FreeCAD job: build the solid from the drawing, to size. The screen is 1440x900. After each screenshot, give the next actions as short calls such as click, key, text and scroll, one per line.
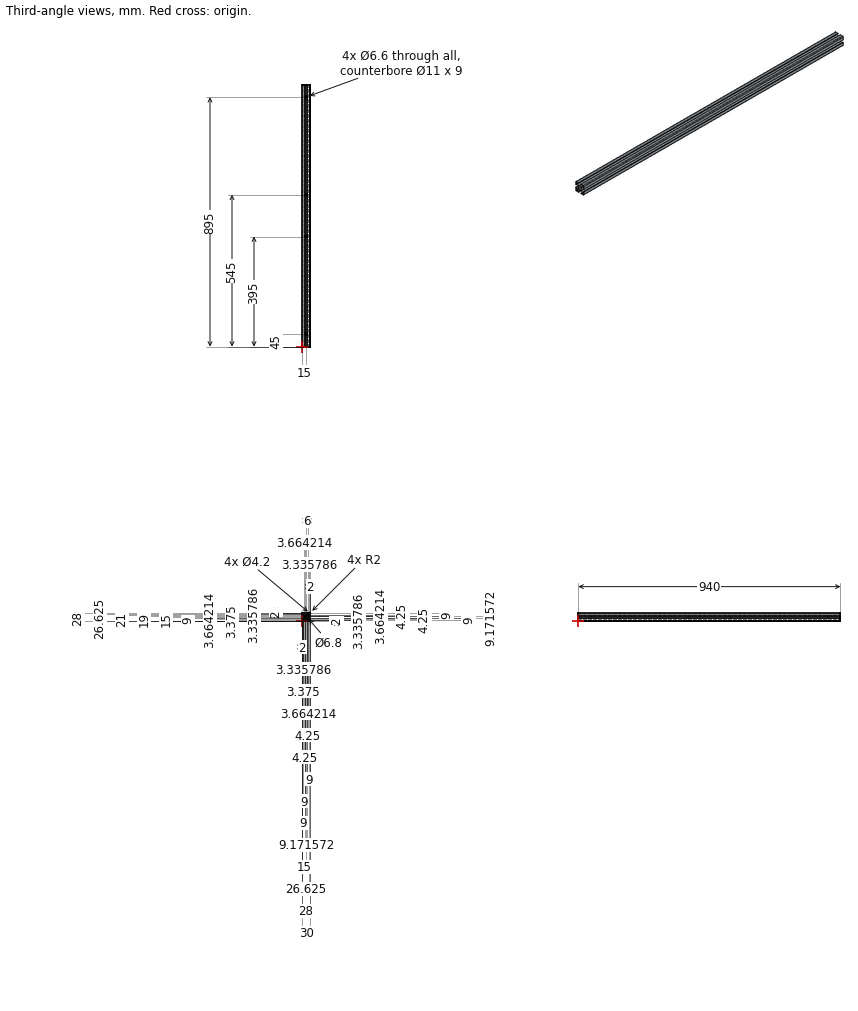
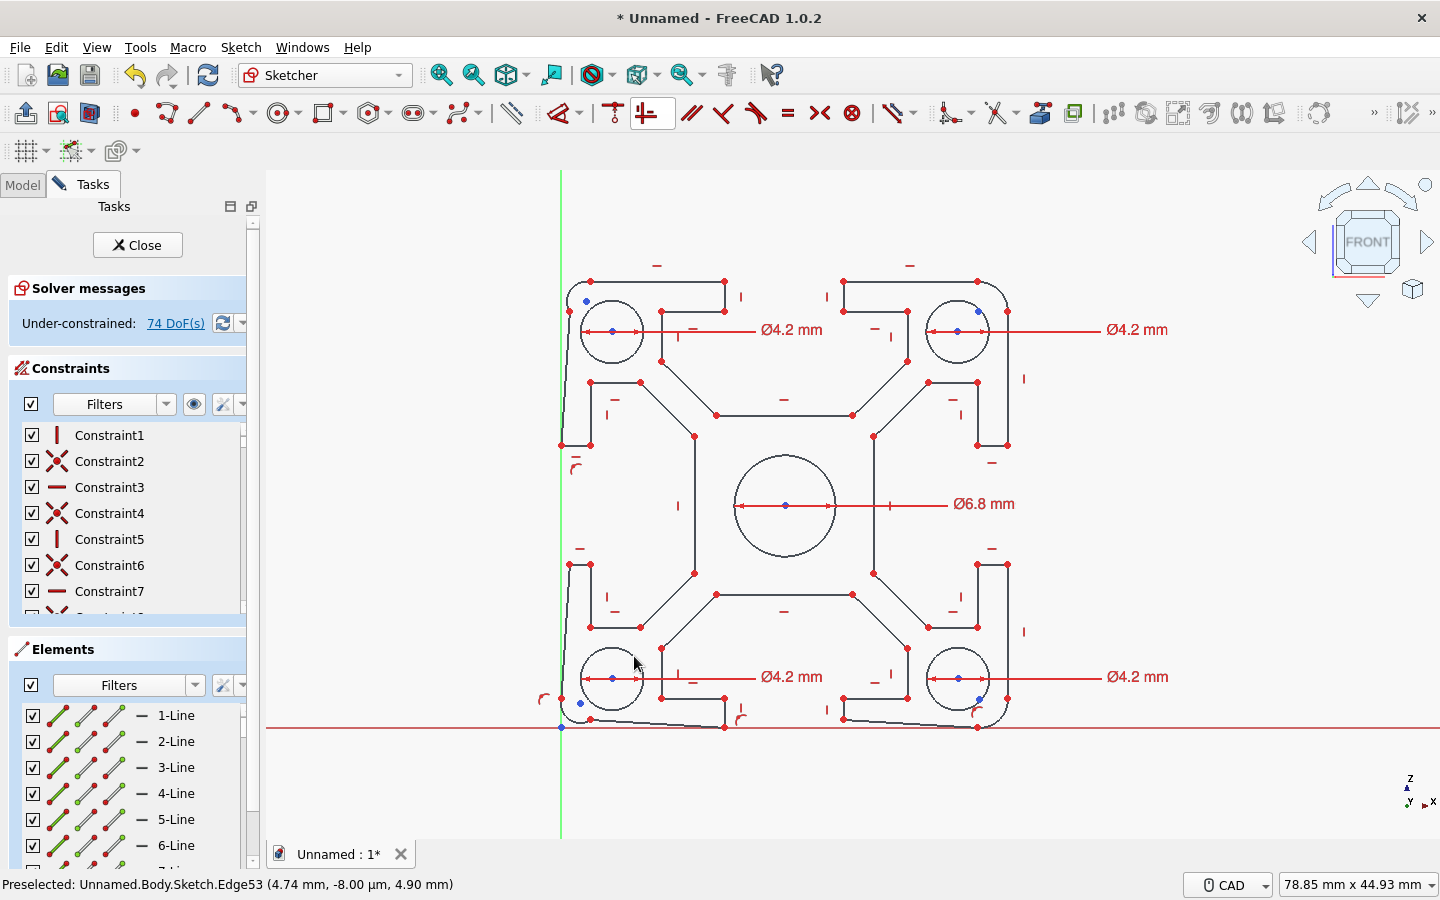
click(1008, 352)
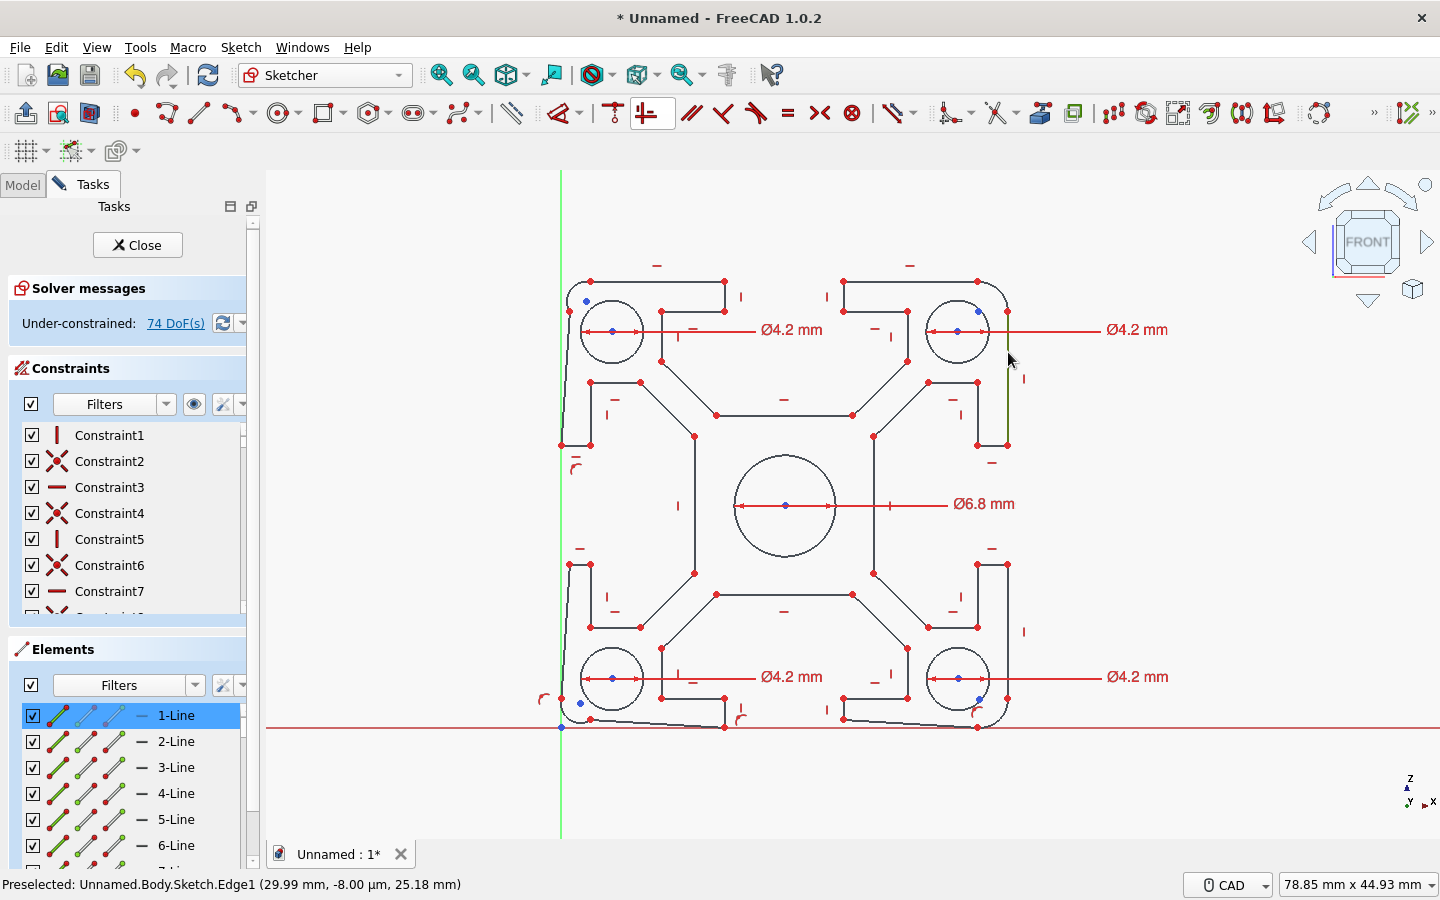
click(1005, 298)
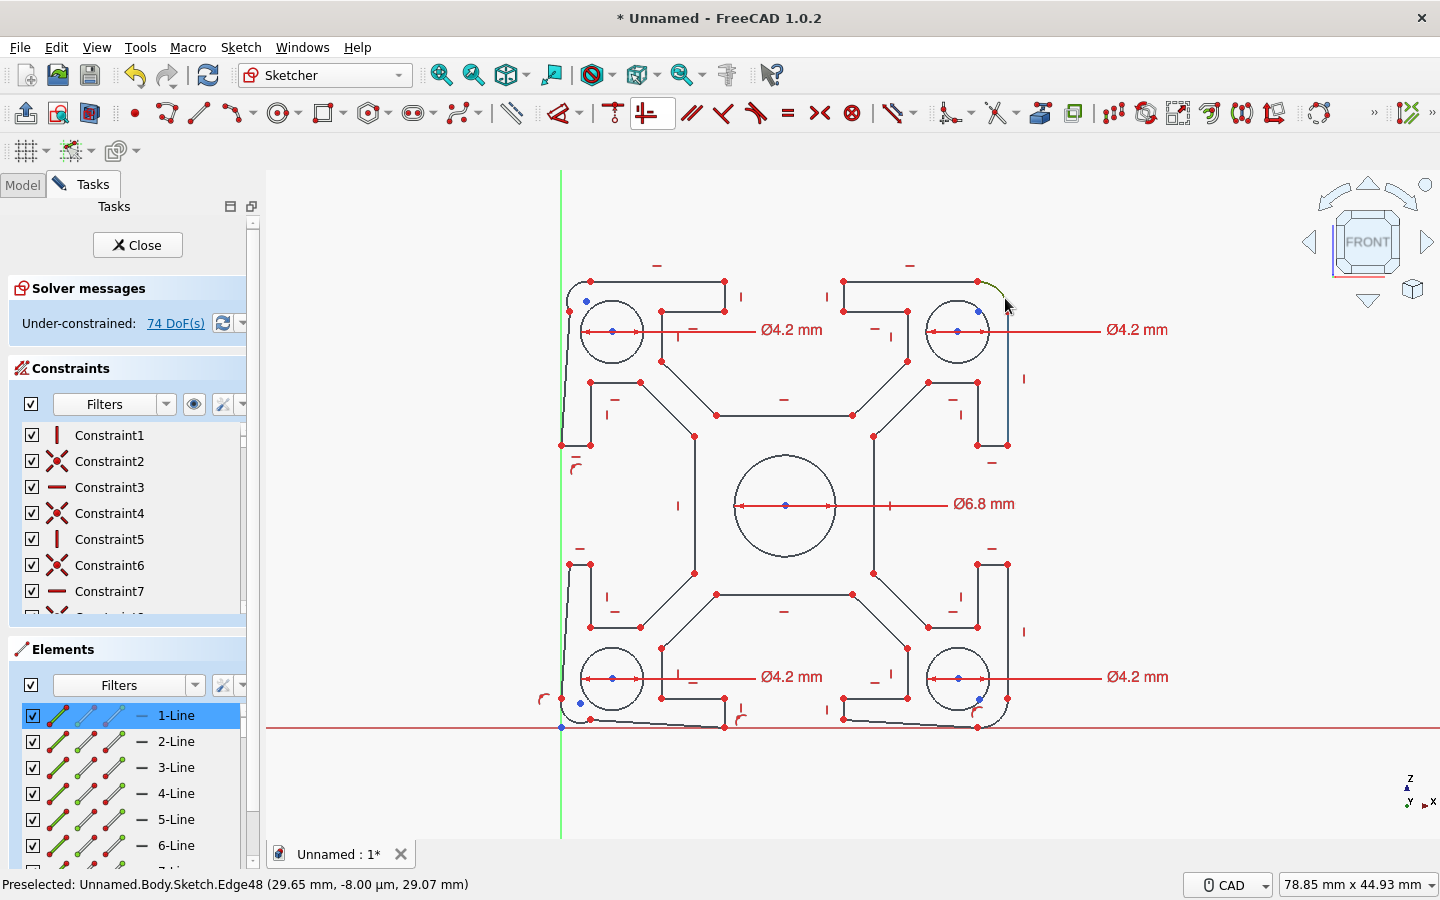
click(756, 114)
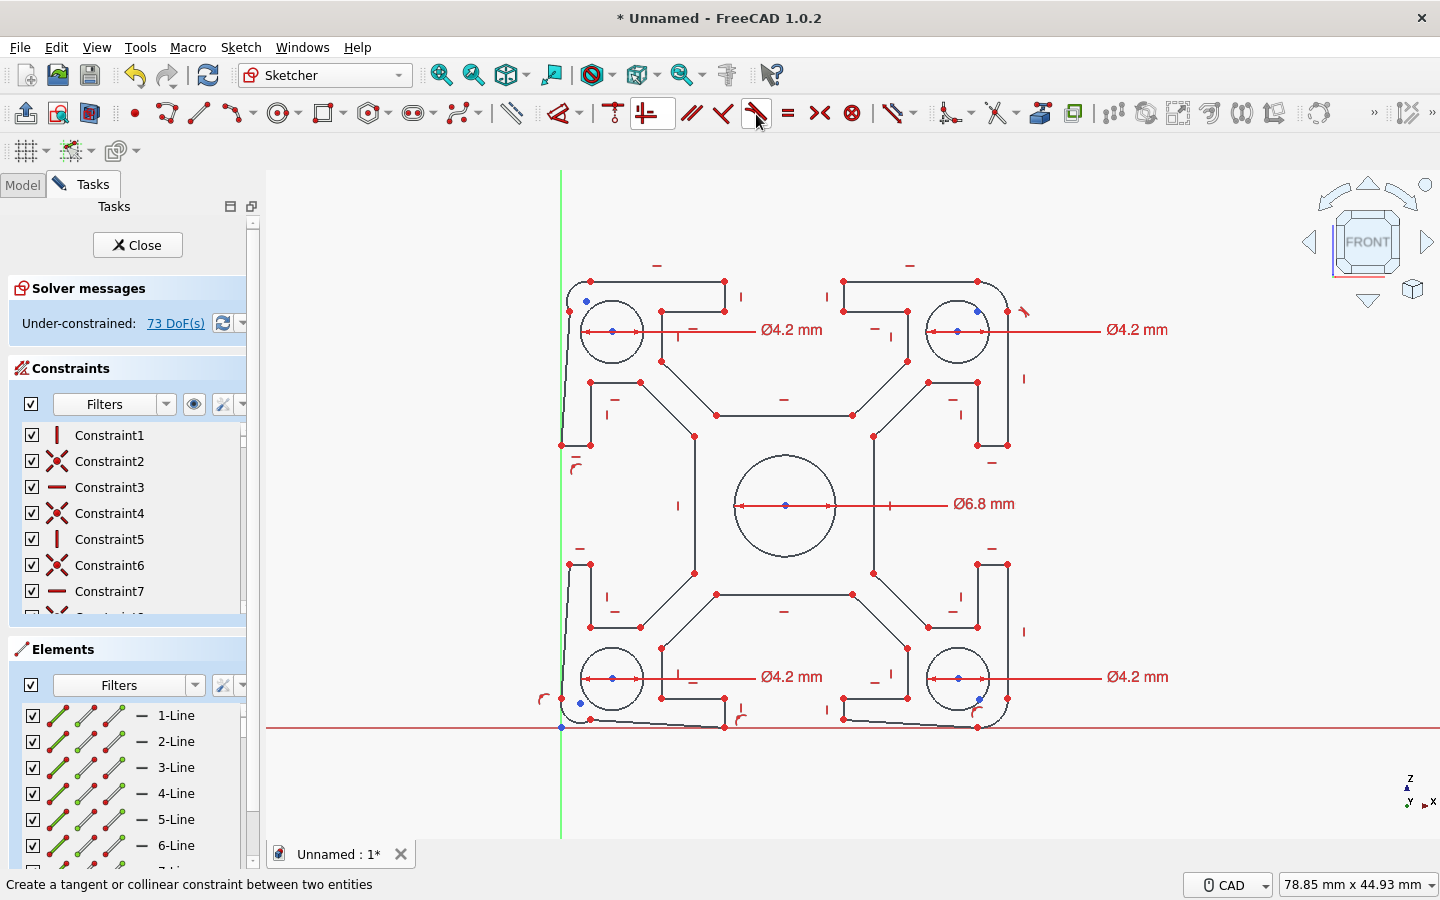
click(1008, 605)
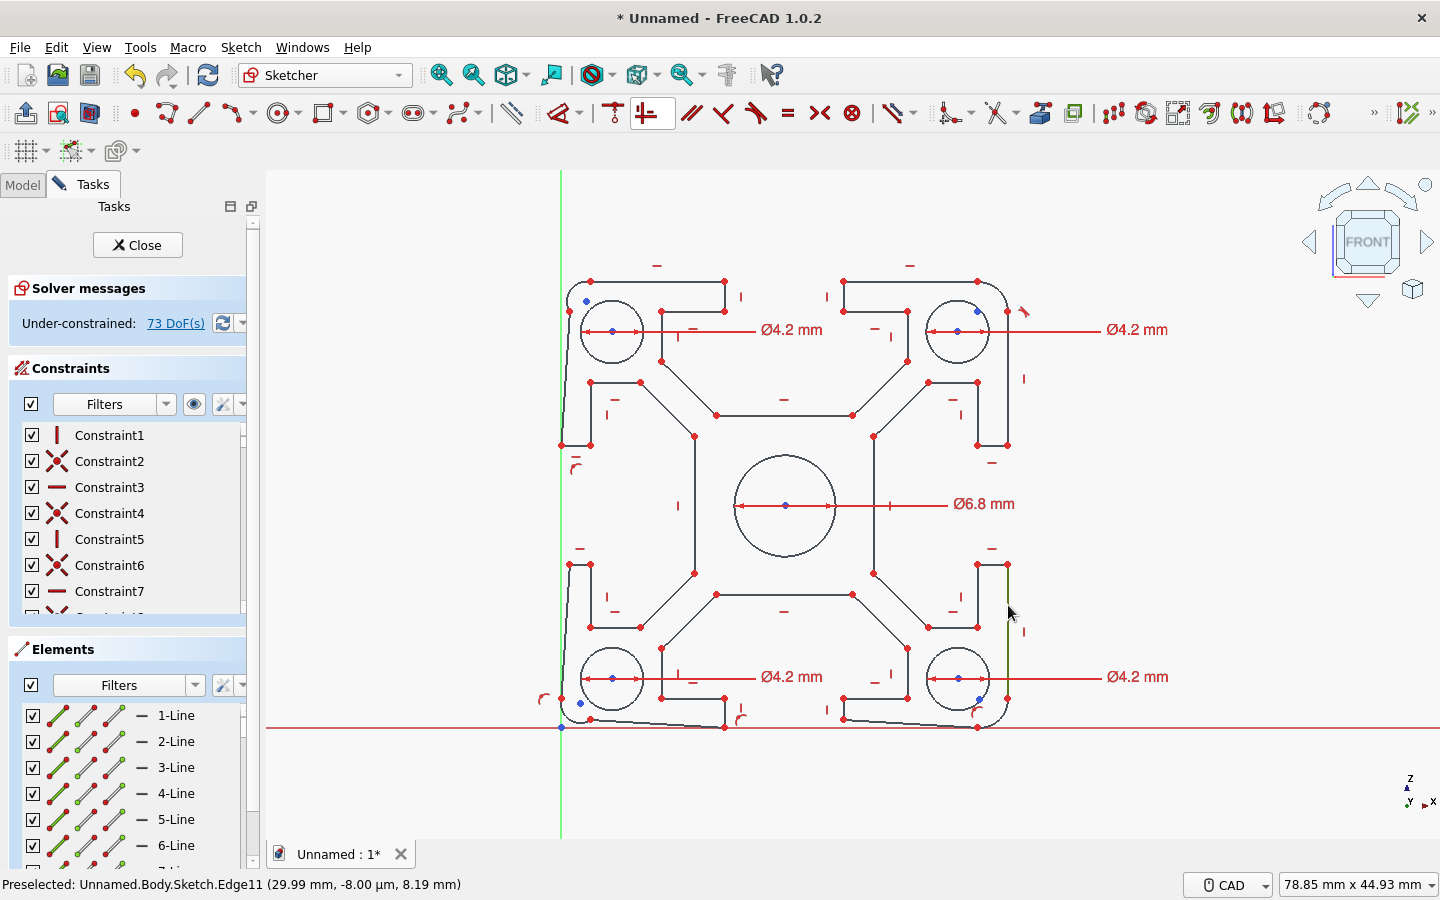
click(992, 725)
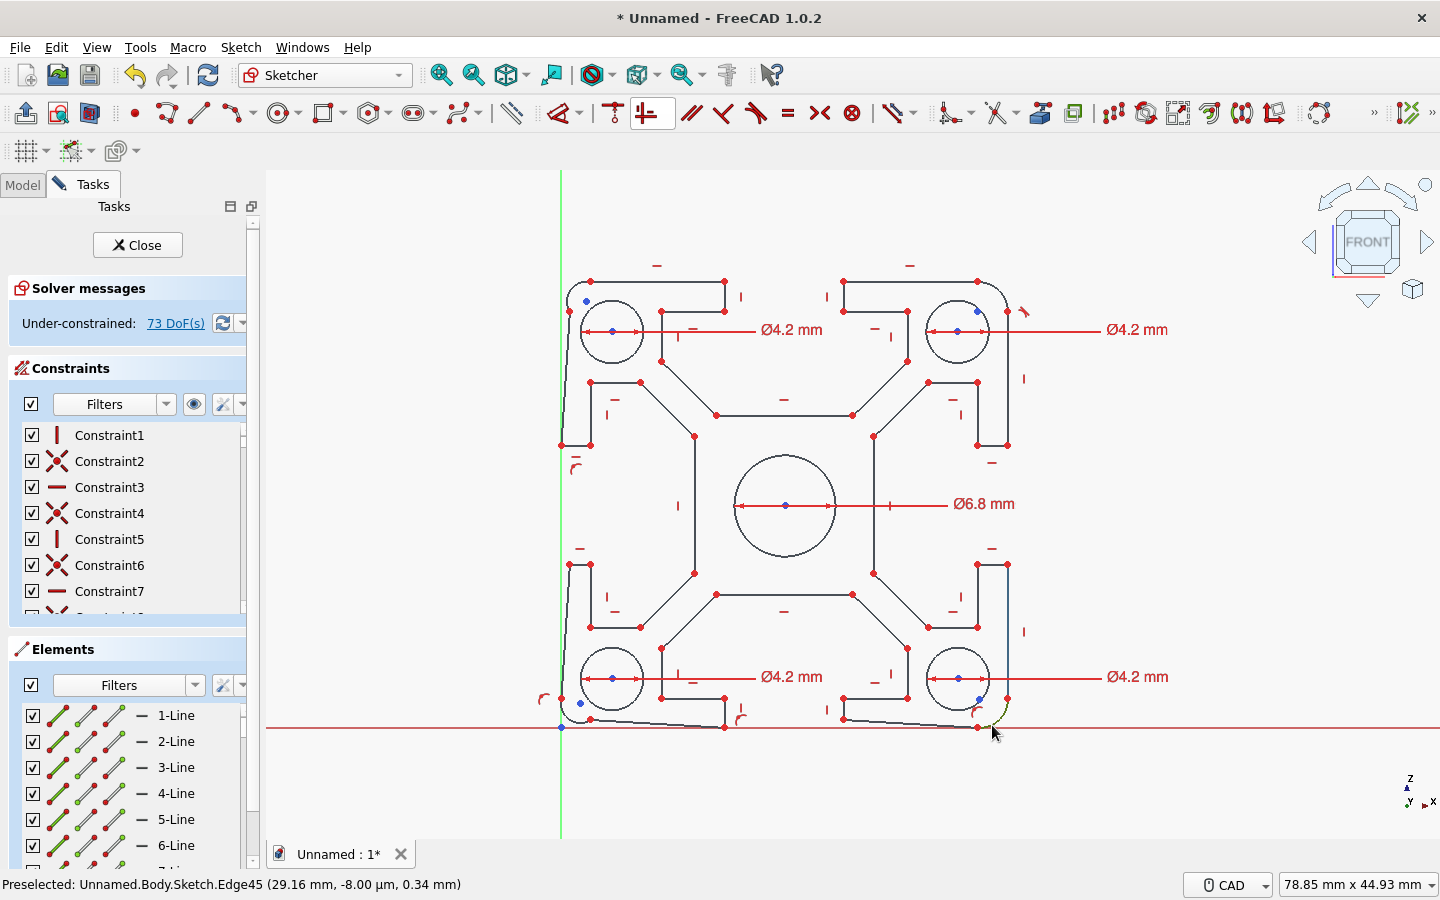
click(756, 114)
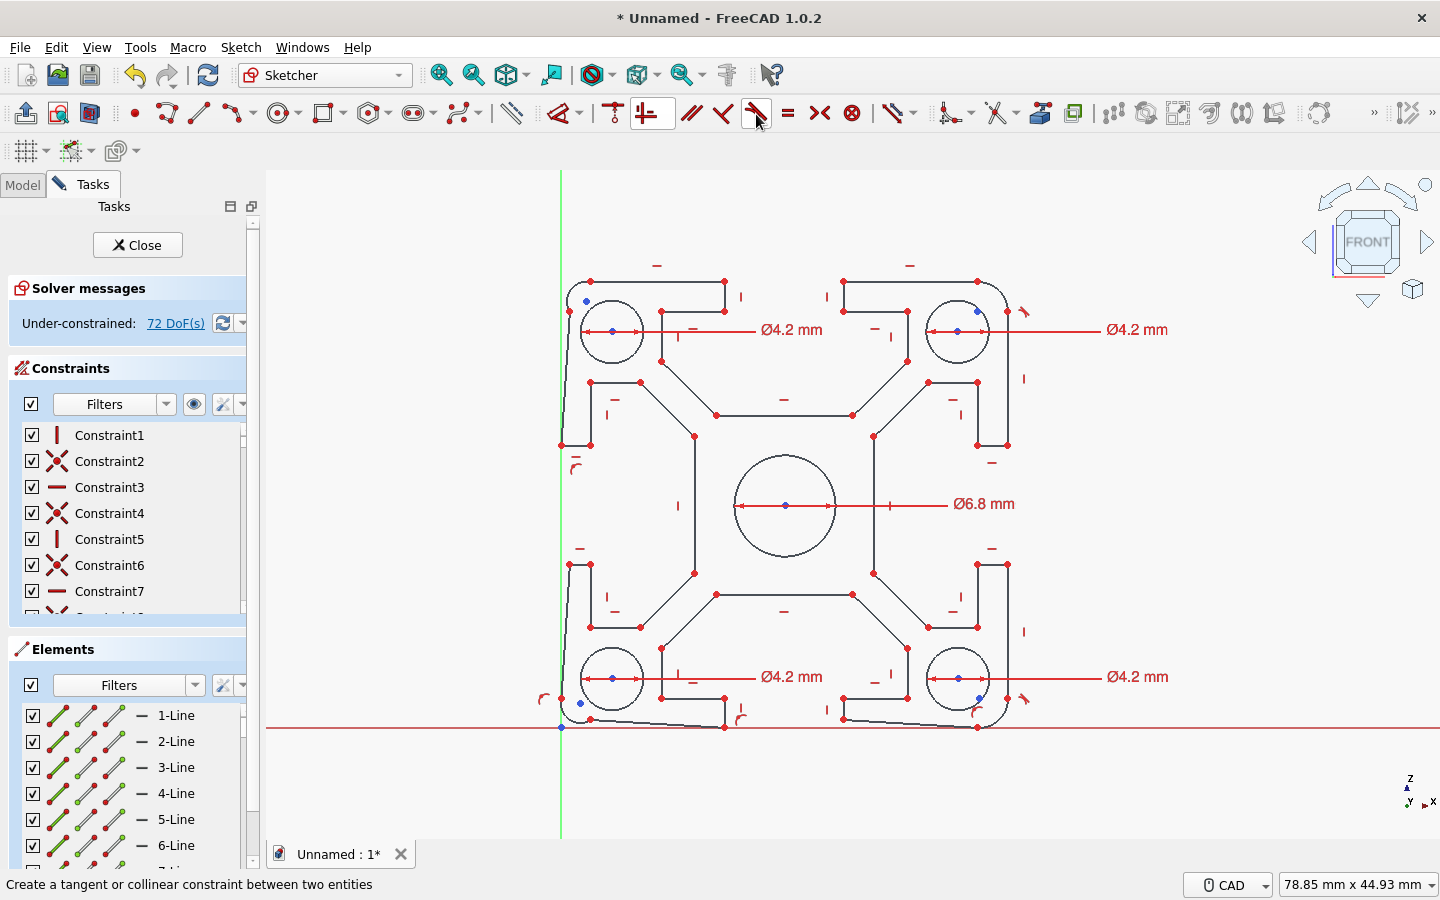
click(938, 726)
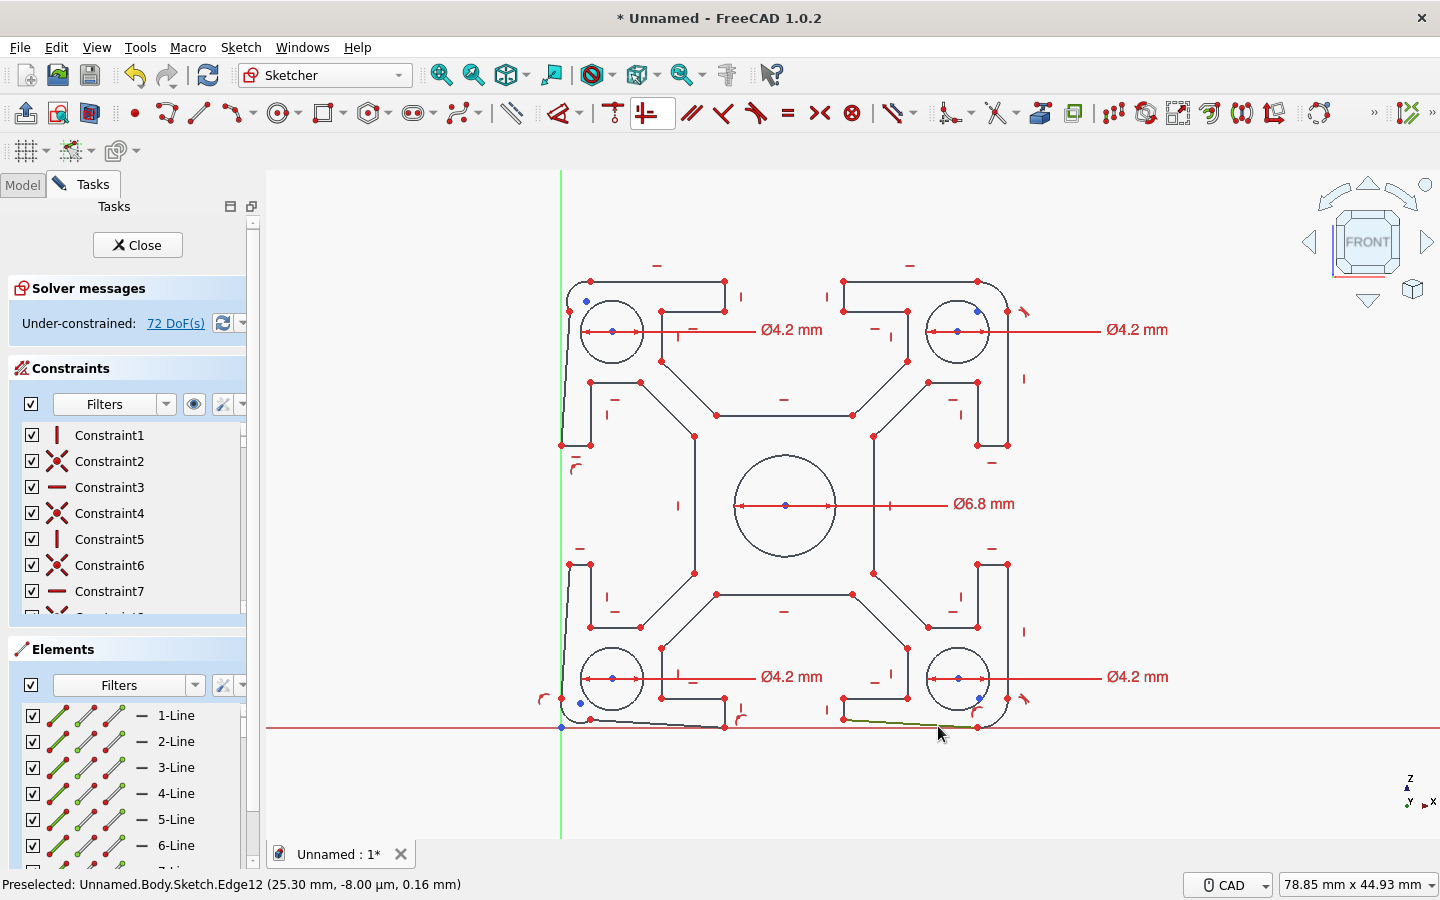
click(991, 725)